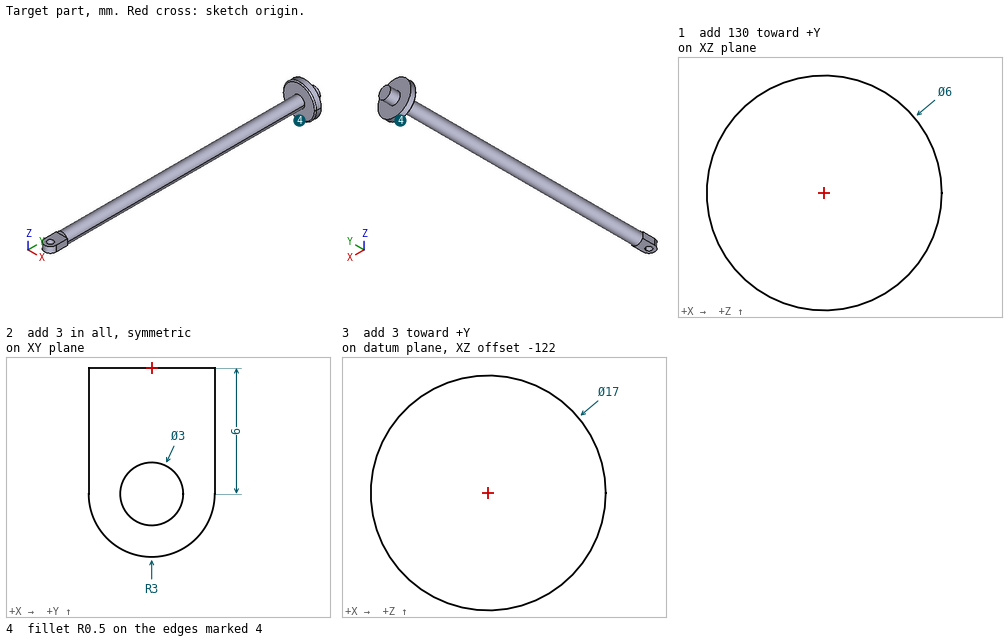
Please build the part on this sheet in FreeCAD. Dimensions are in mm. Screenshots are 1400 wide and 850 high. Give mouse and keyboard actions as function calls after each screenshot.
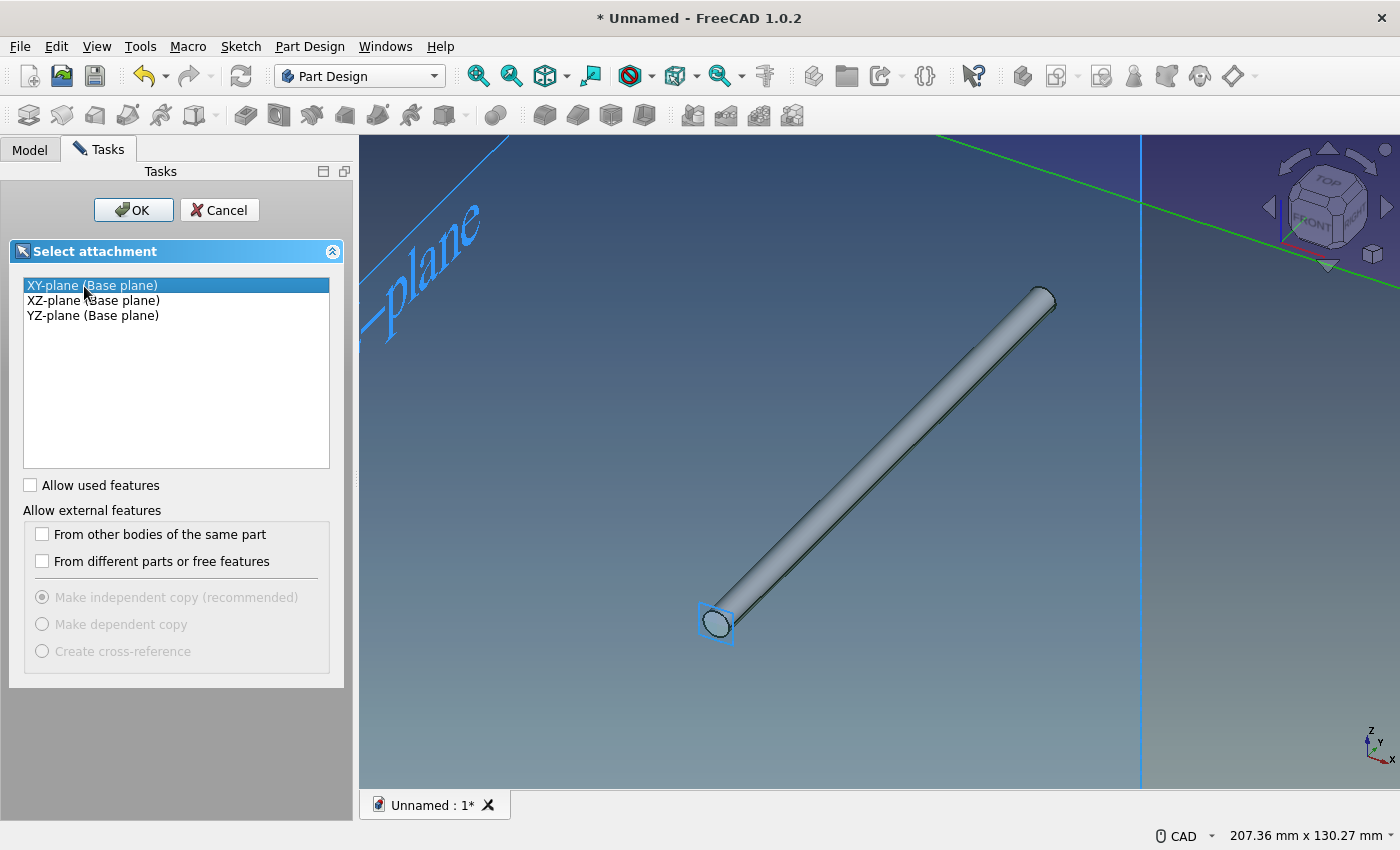
click(134, 210)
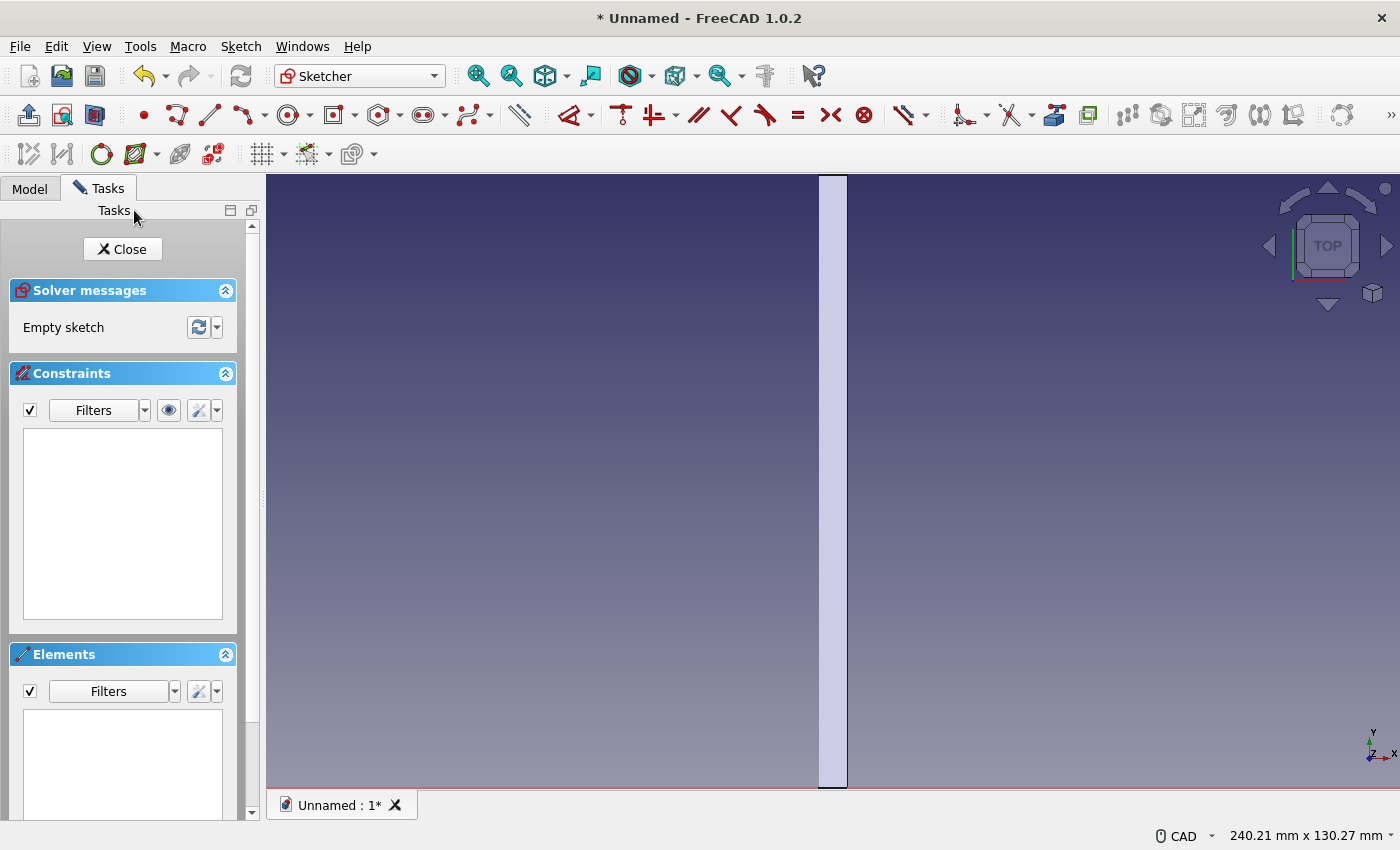
key(q)
key(s)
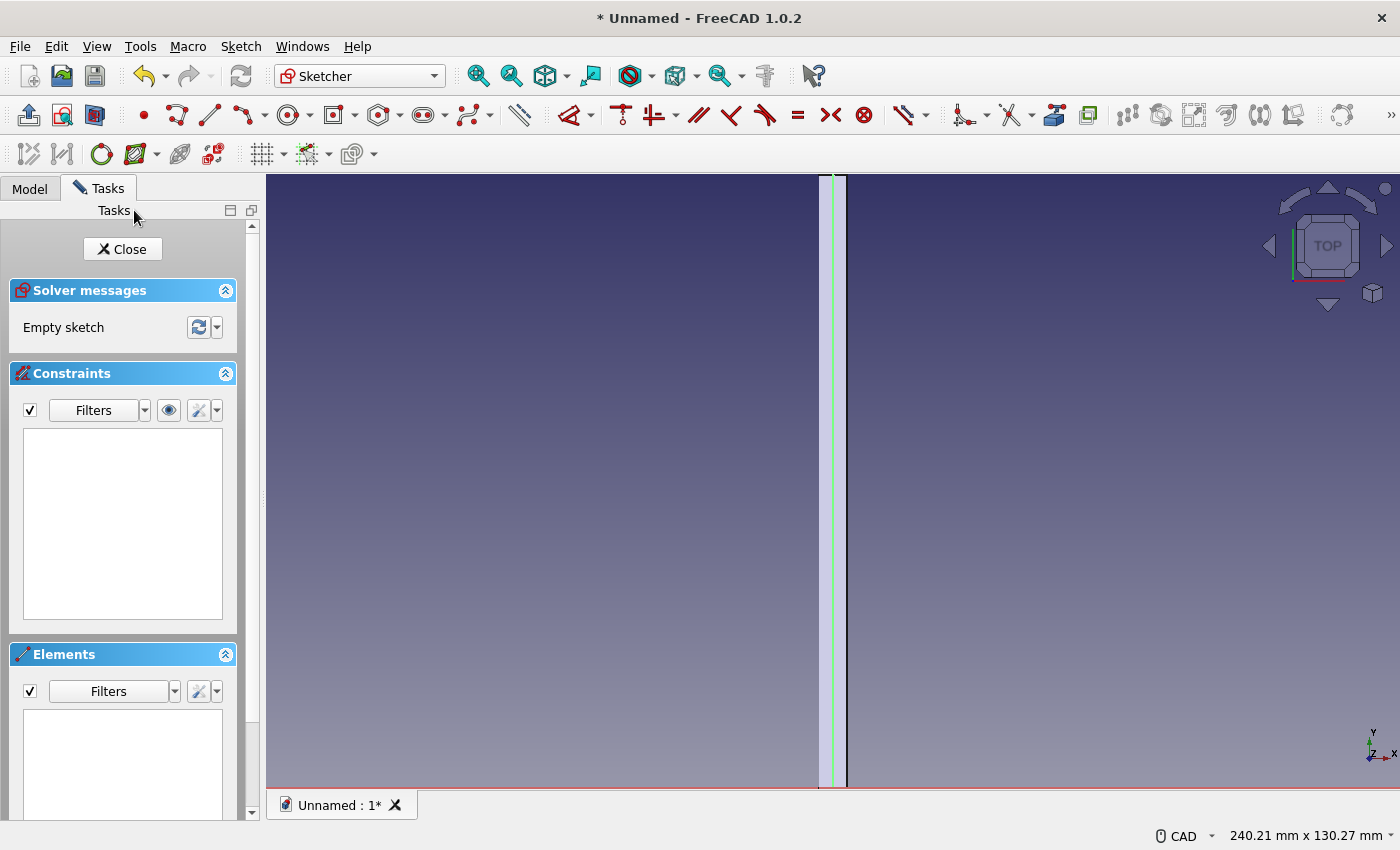
scroll(764, 482, down, 5)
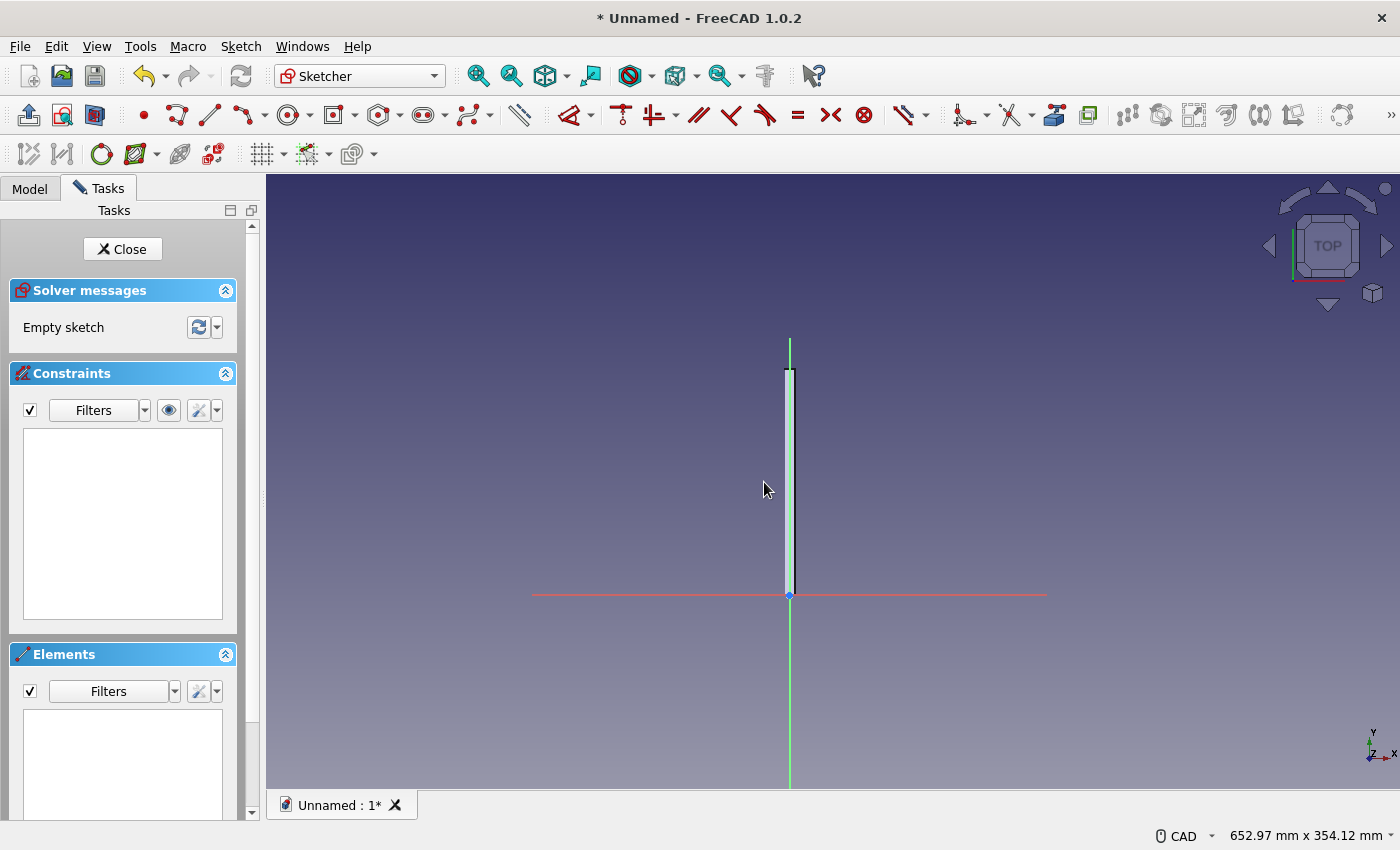
scroll(791, 609, up, 15)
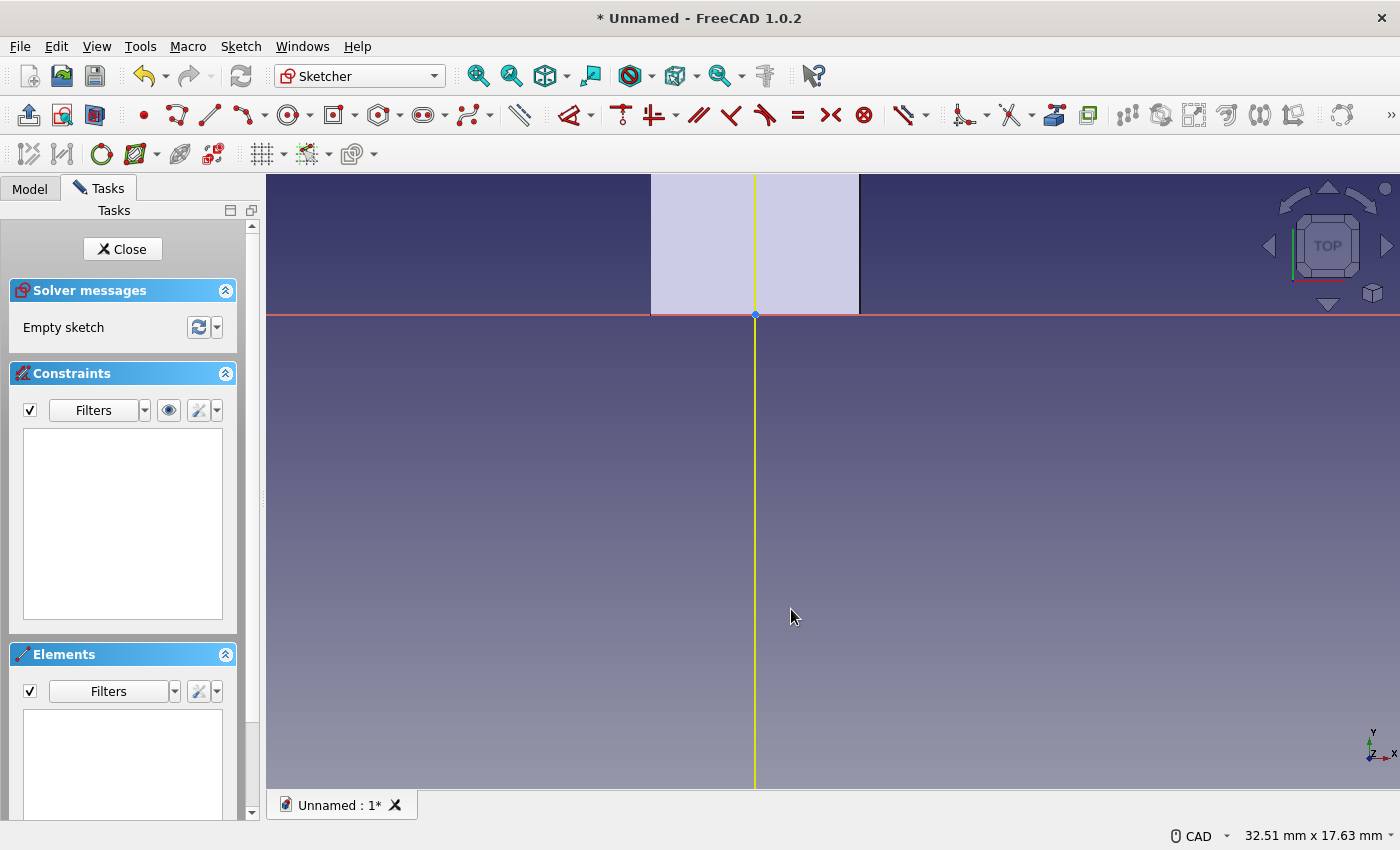
key(g)
key(m)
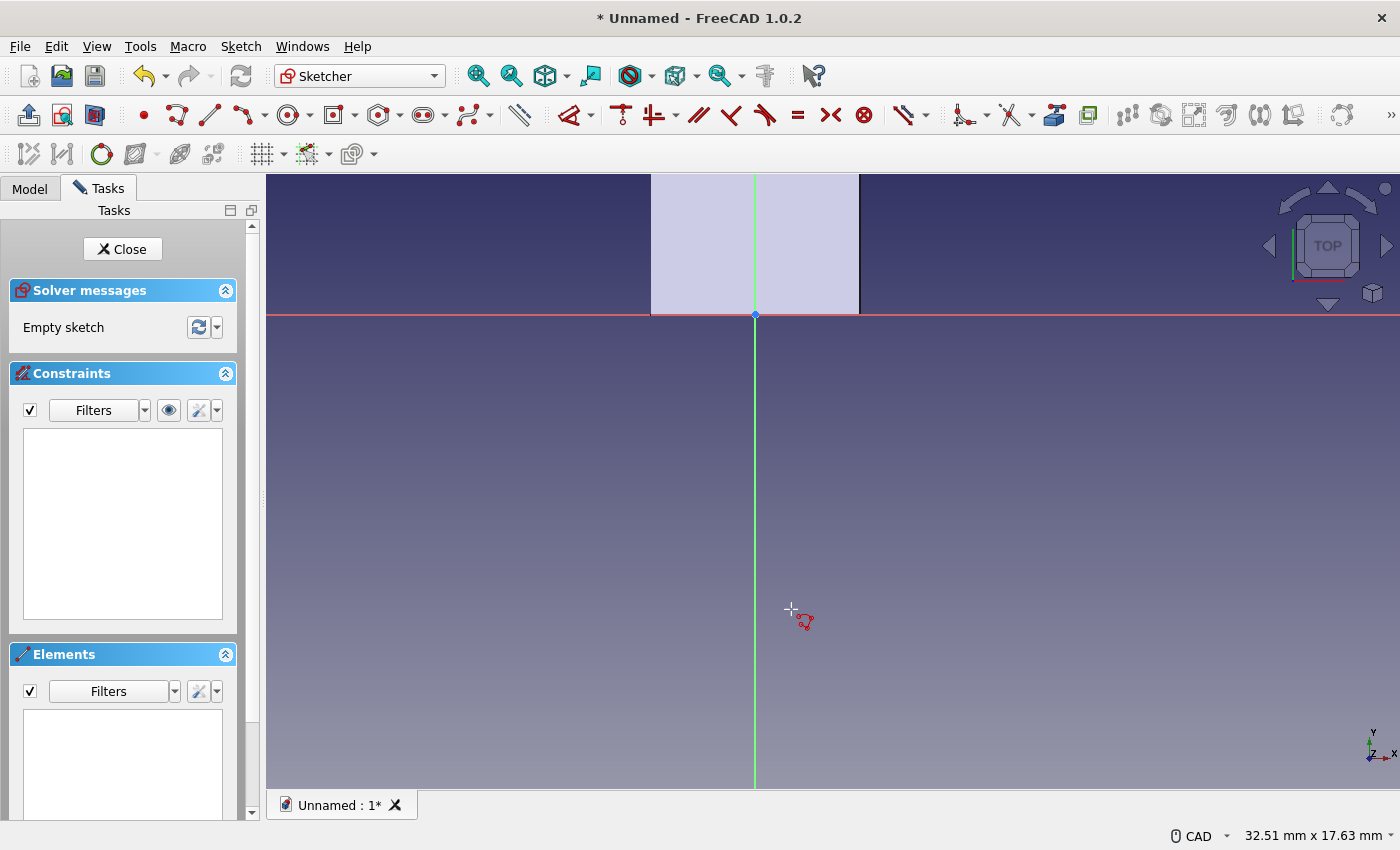
click(860, 524)
click(860, 315)
click(651, 324)
click(651, 524)
right_click(651, 524)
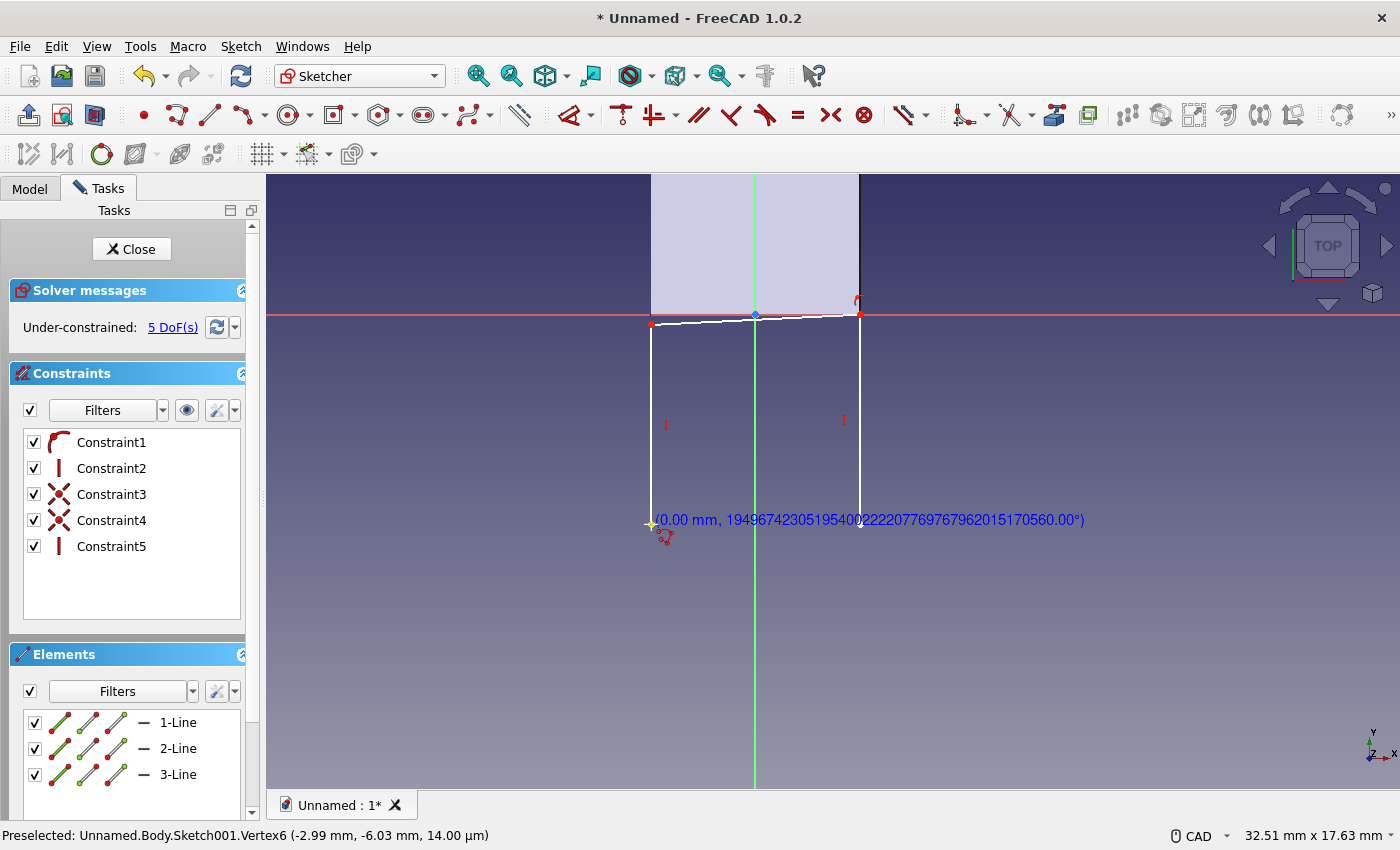
key(g)
key(3)
key(a)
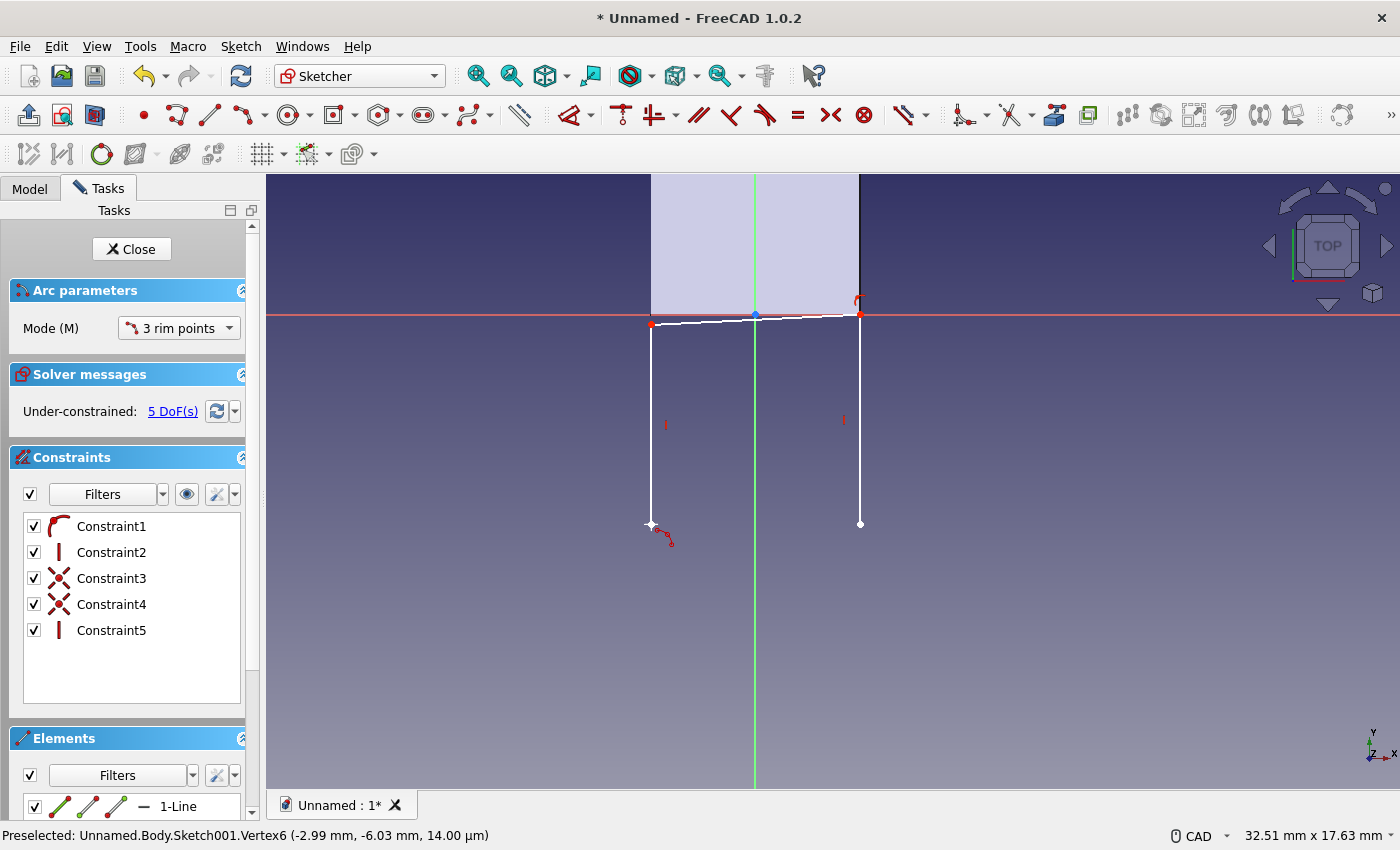
click(651, 525)
click(860, 525)
click(723, 623)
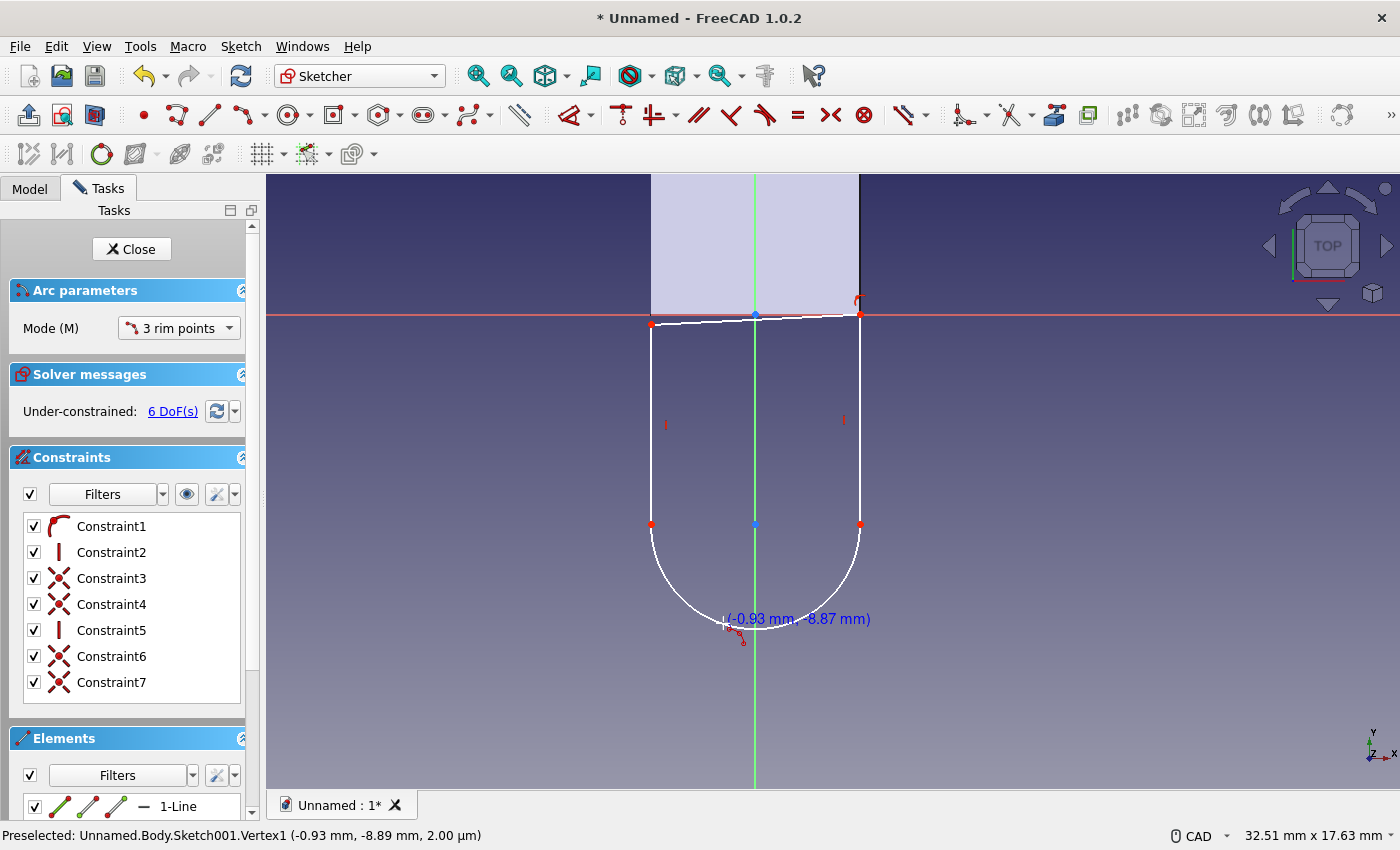
key(g)
key(c)